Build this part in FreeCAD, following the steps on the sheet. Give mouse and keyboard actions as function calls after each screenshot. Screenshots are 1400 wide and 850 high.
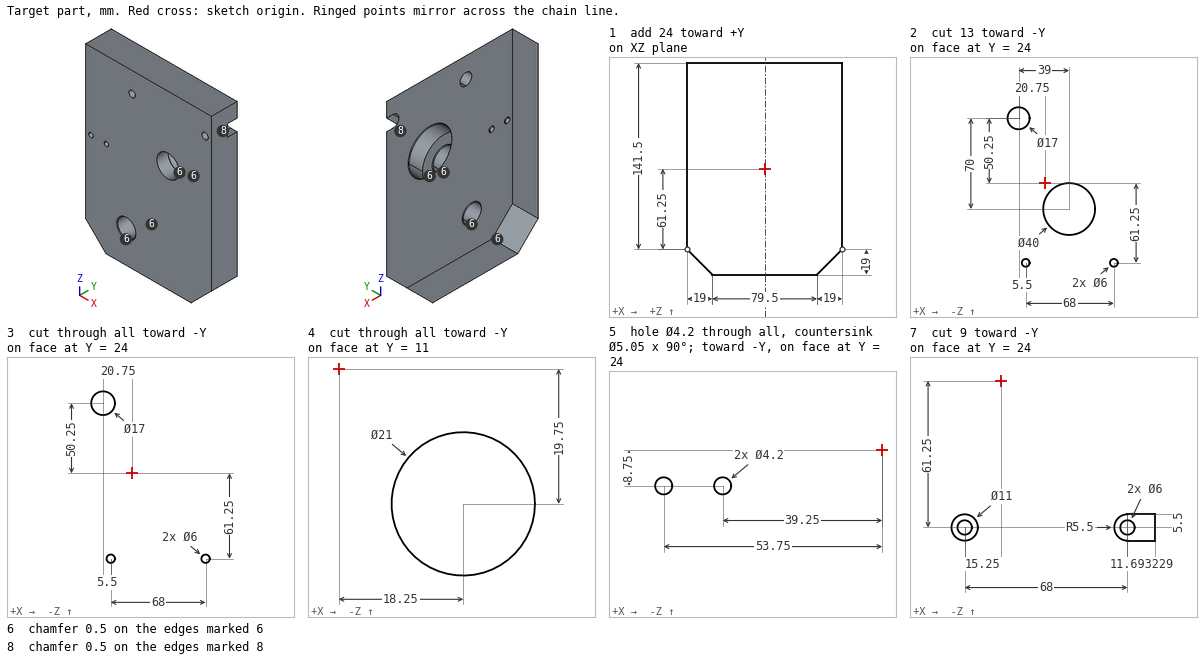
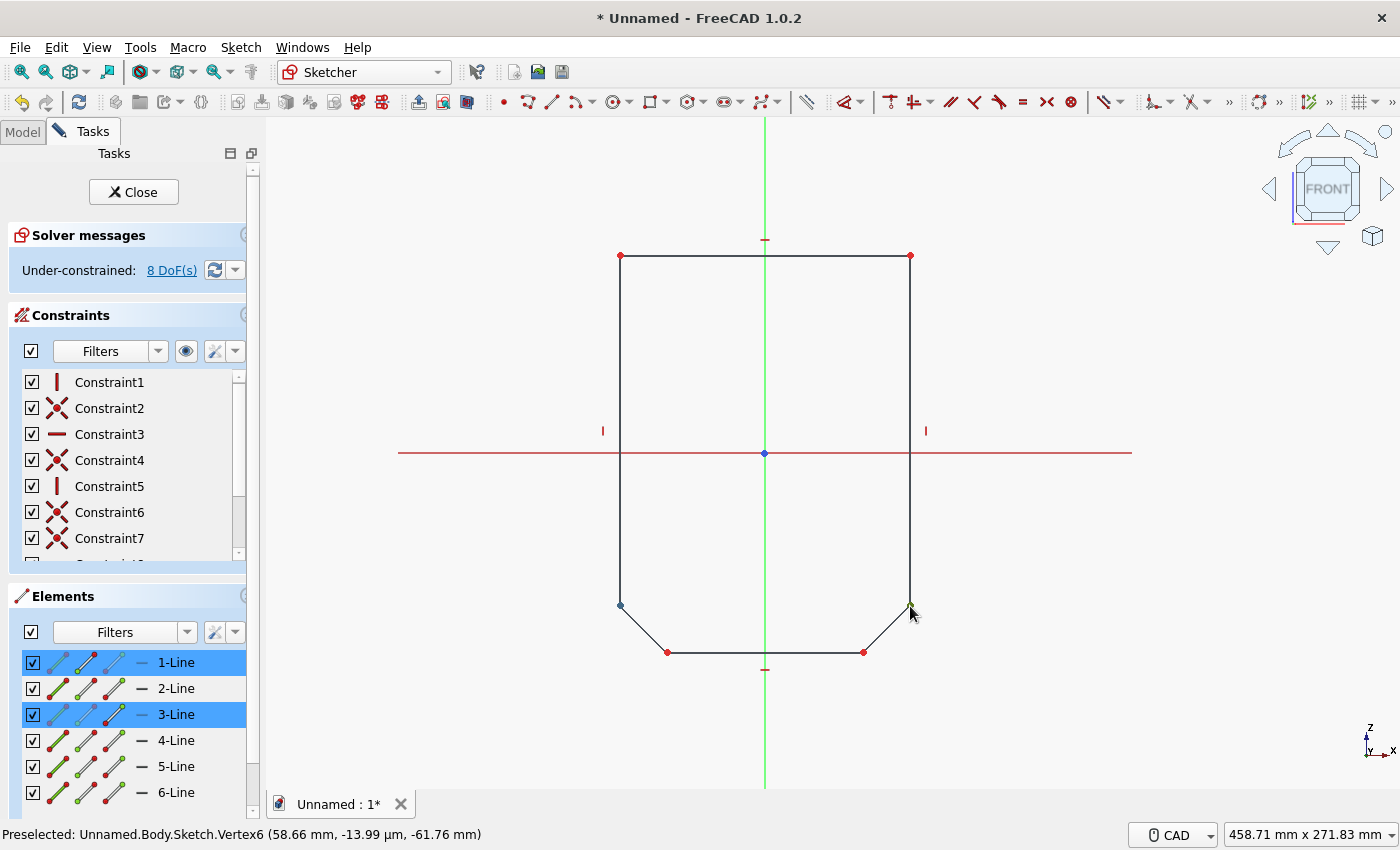
click(765, 717)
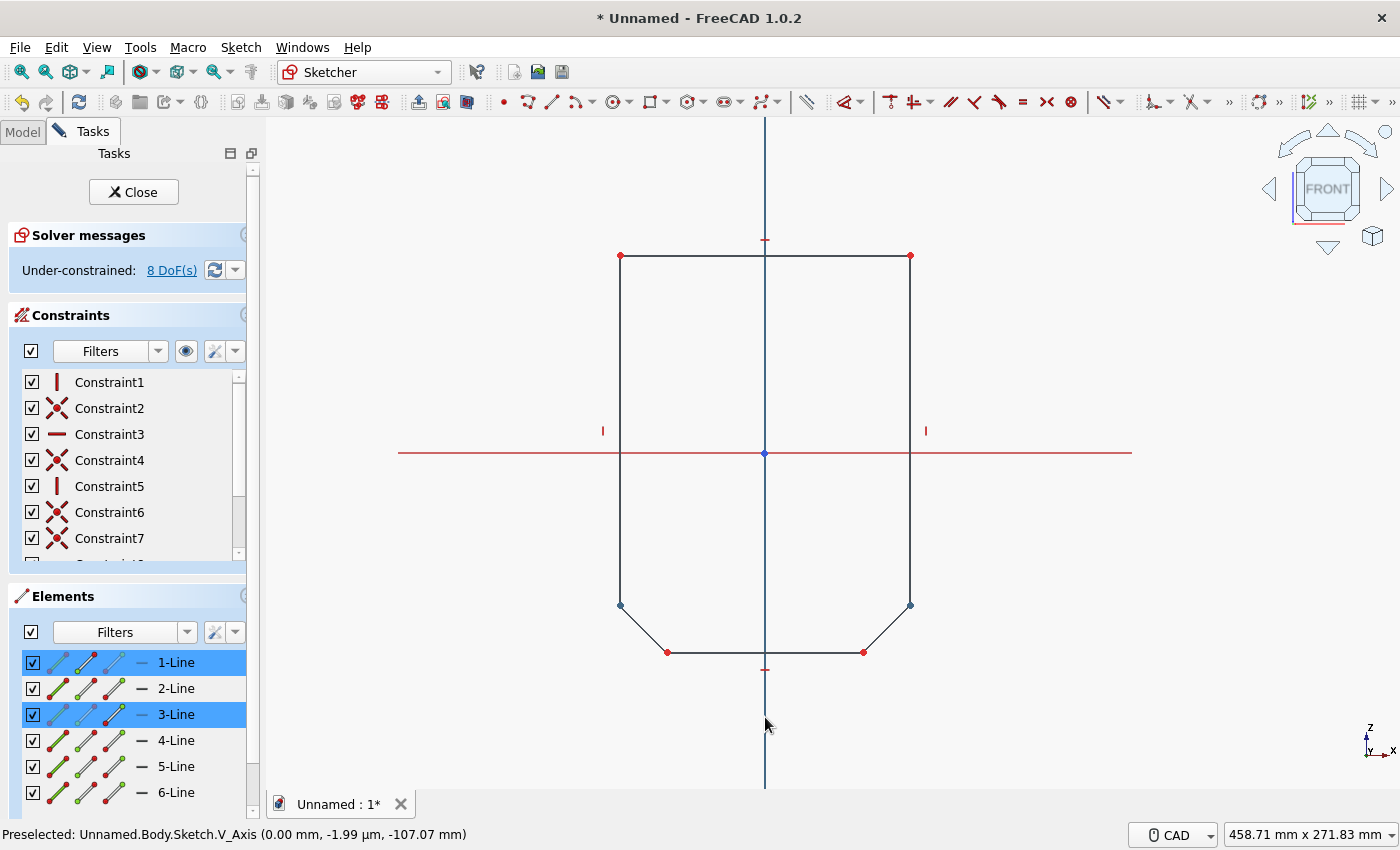
key(s)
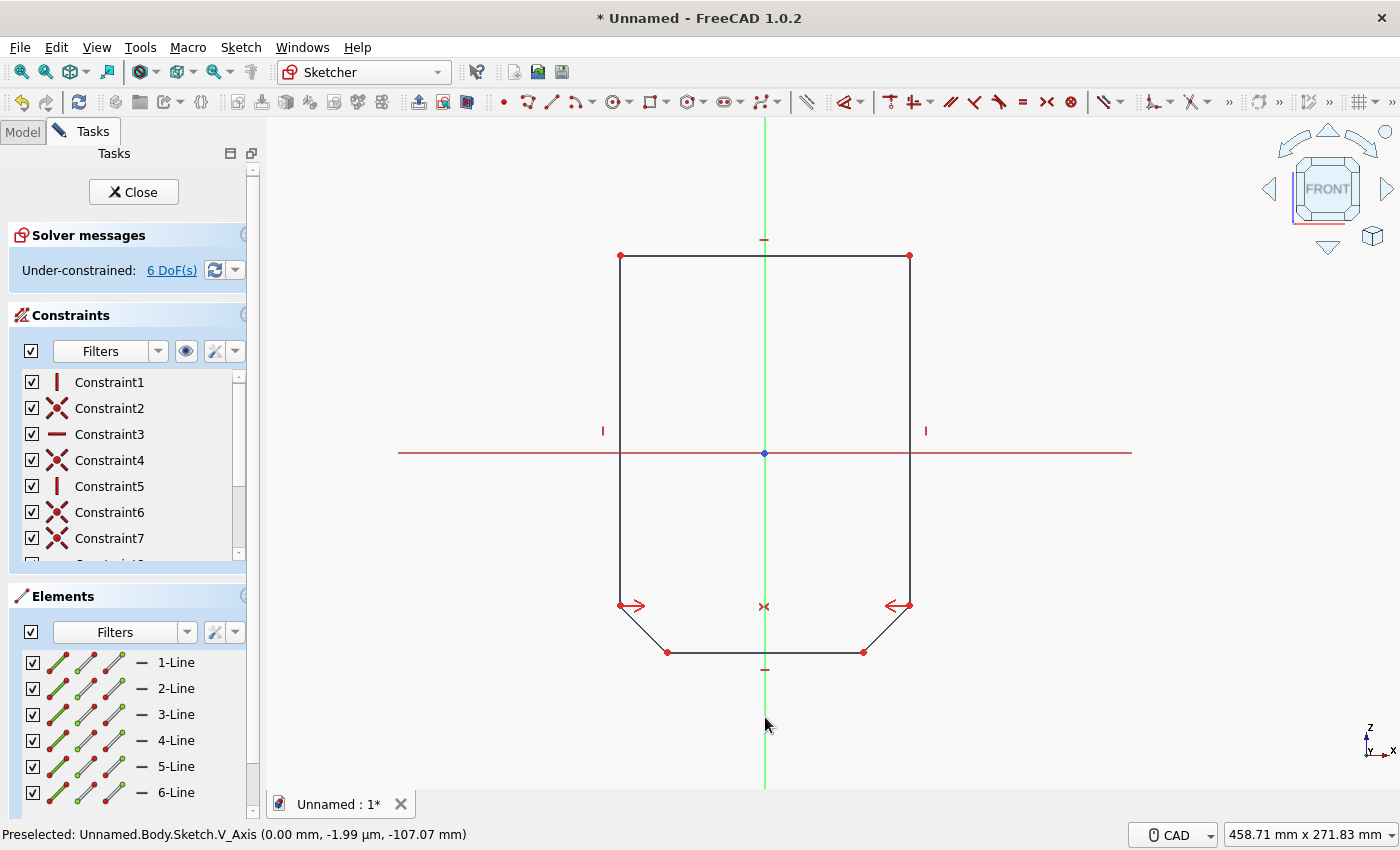
key(d)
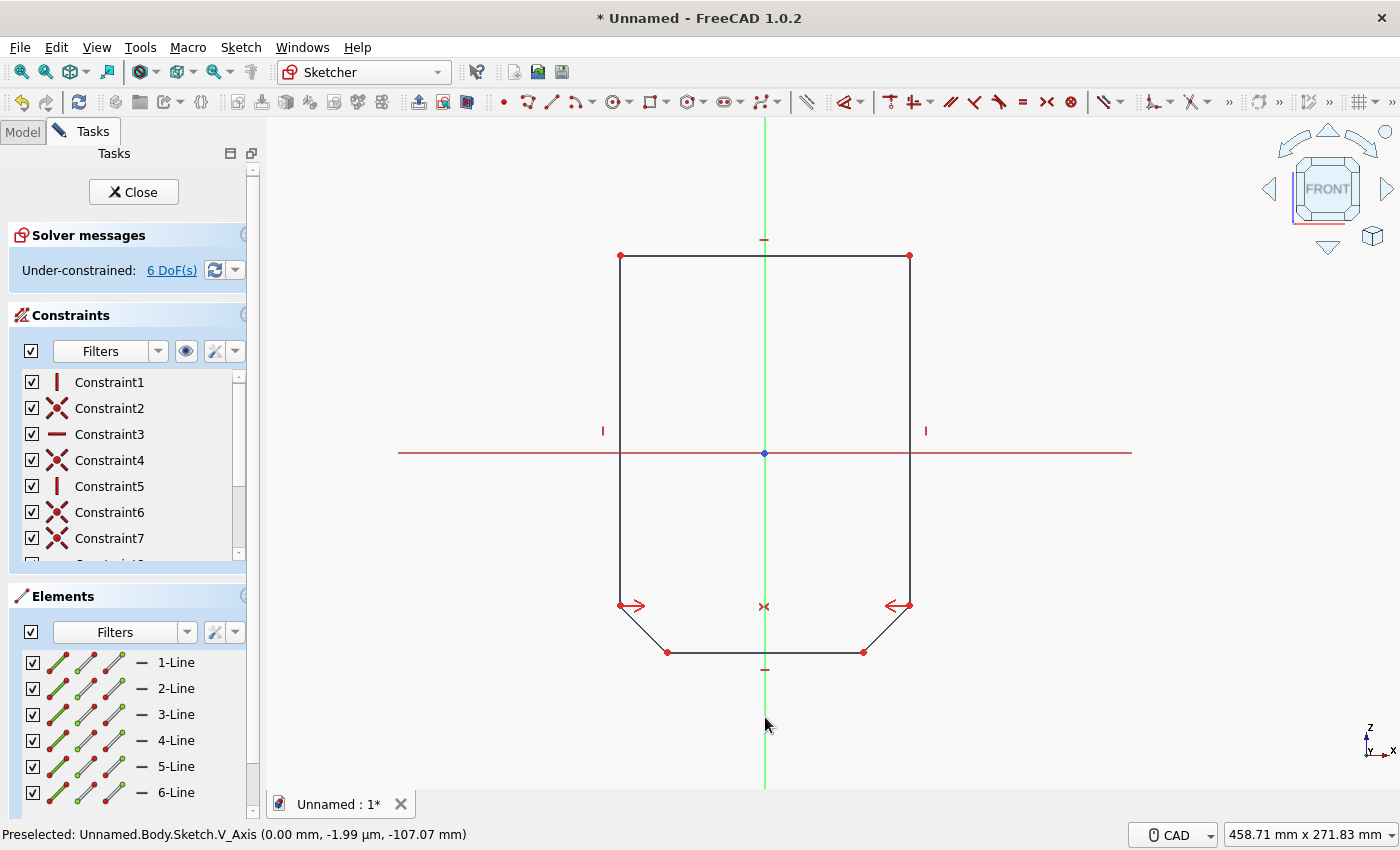
click(896, 620)
click(886, 687)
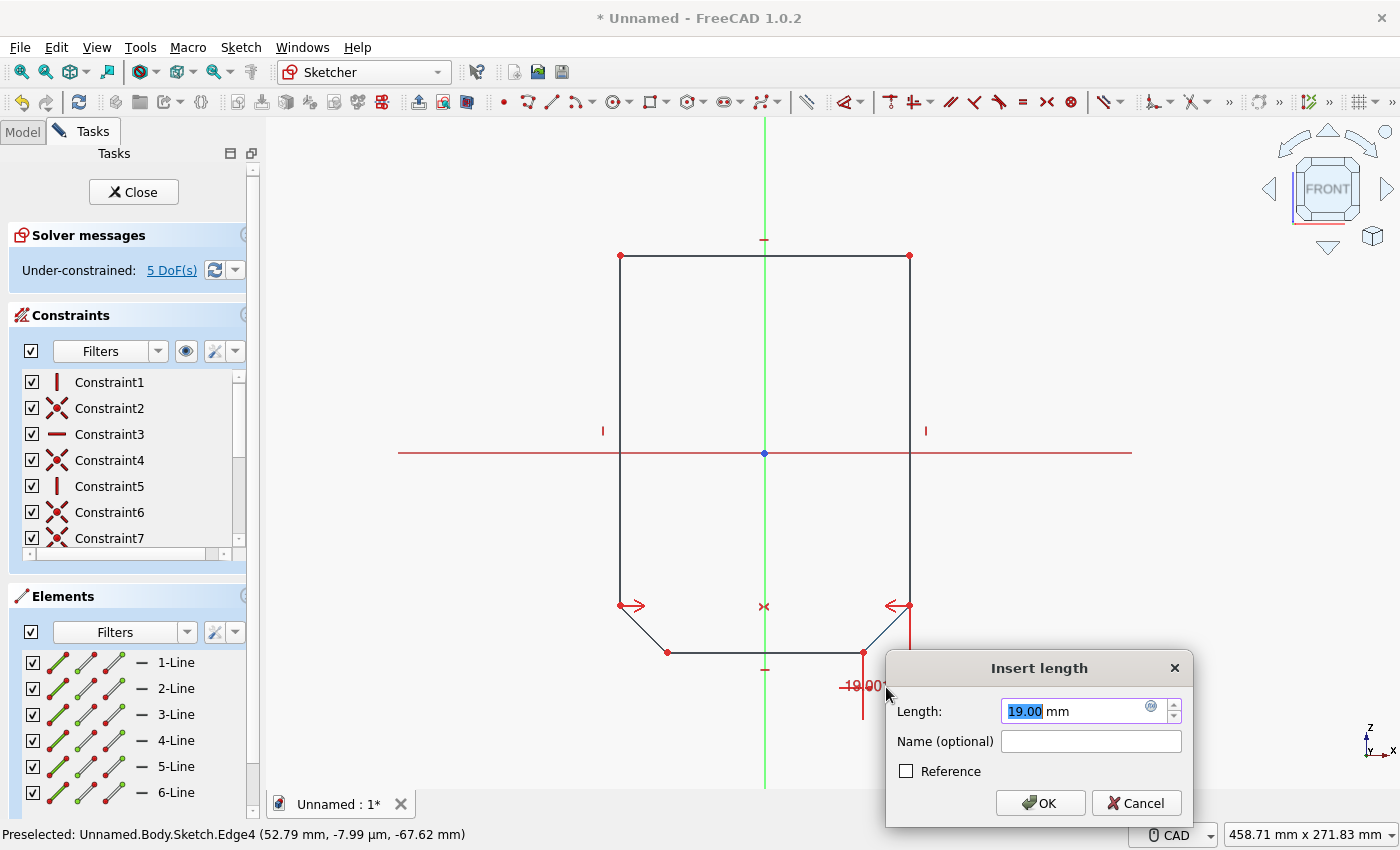
text(19)
key(Return)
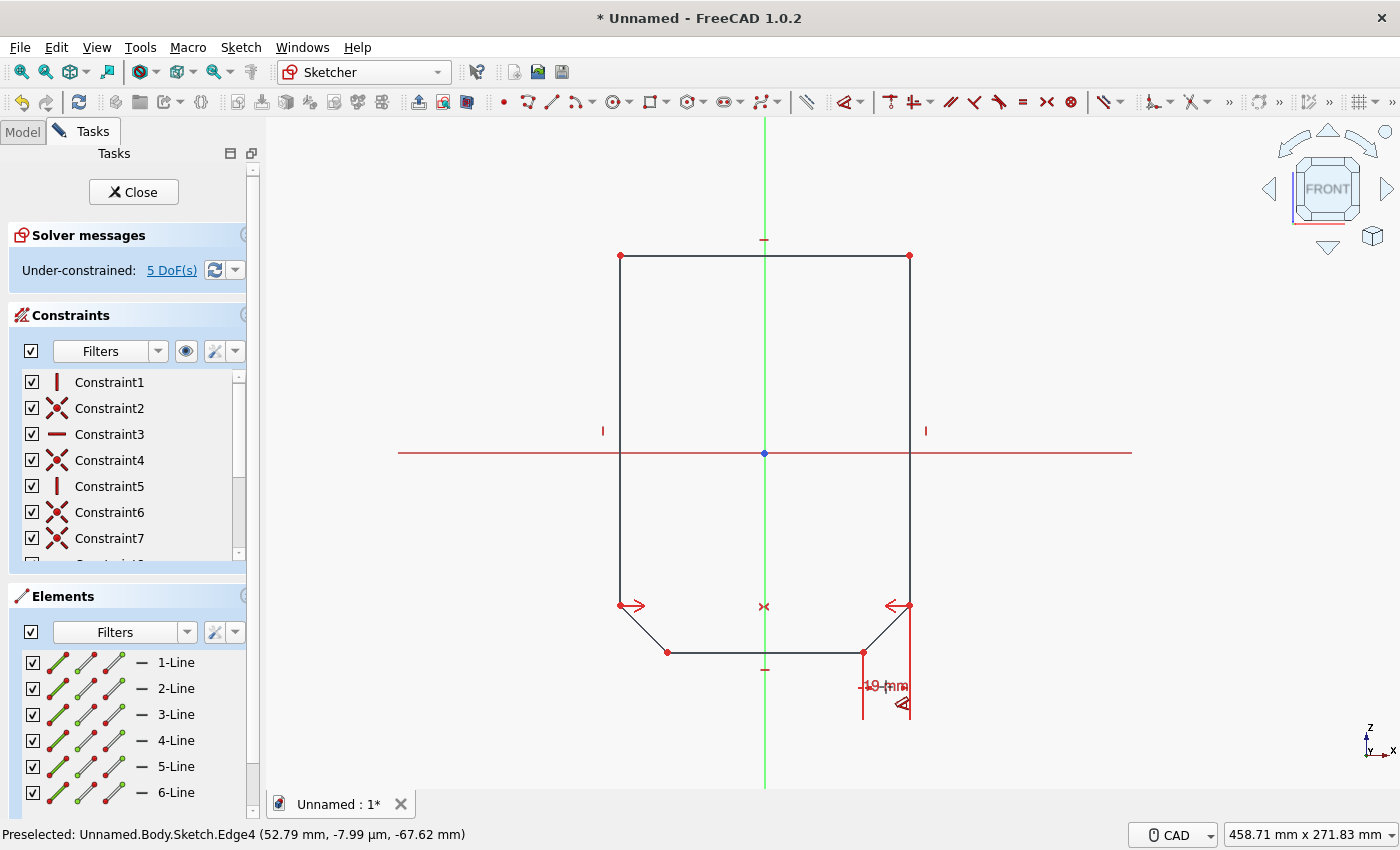
click(896, 620)
click(944, 629)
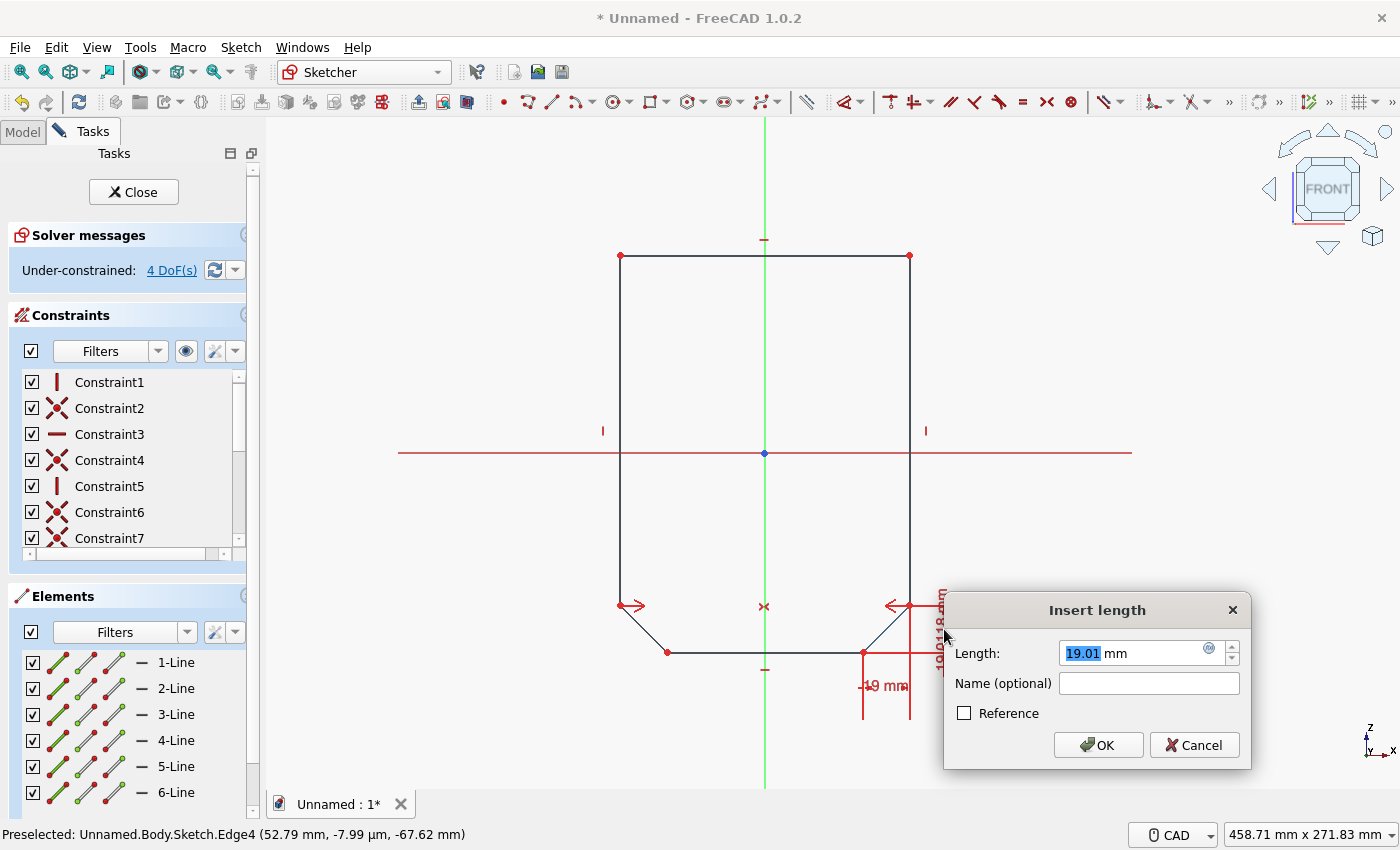
text(19)
key(Return)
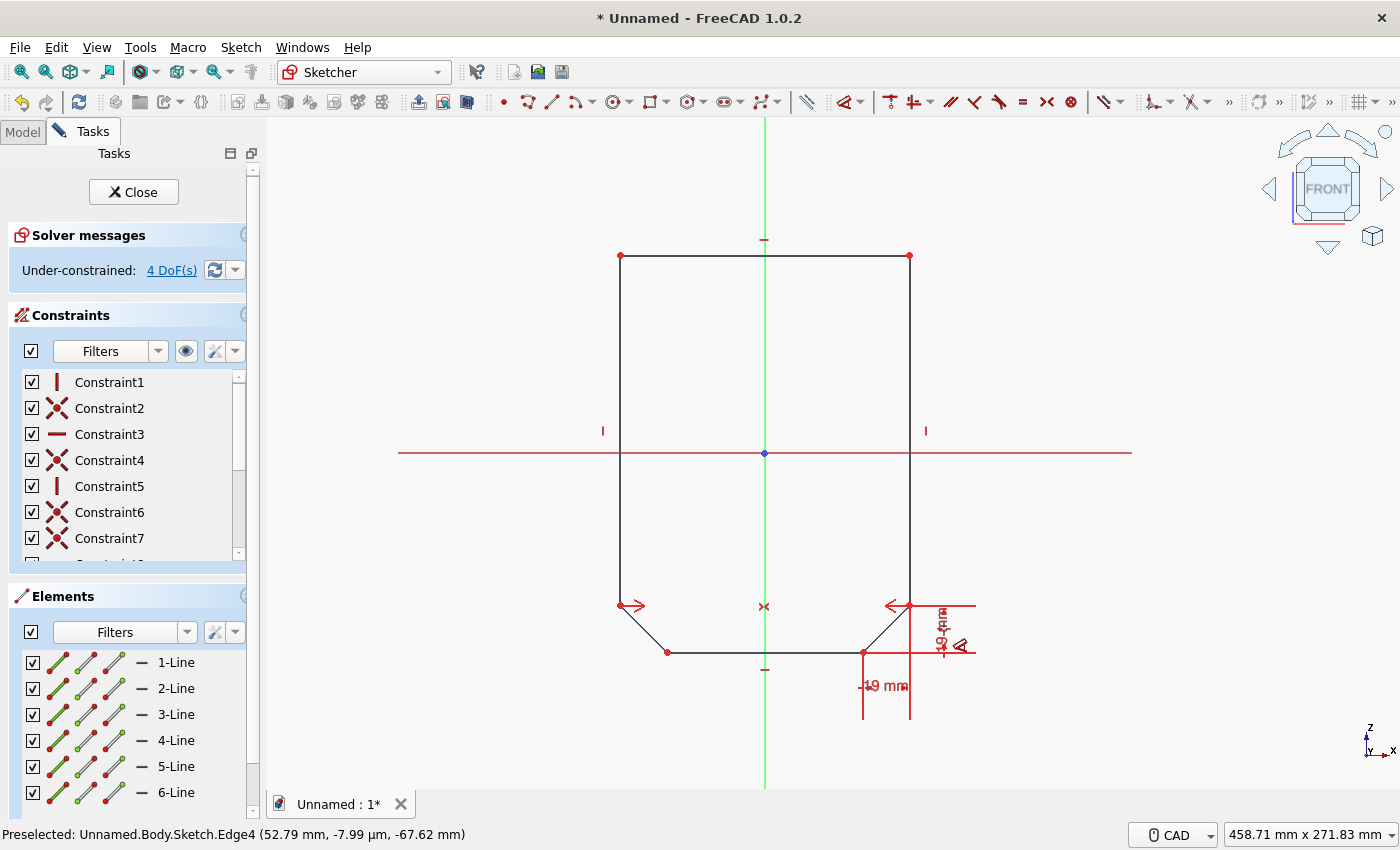
click(653, 639)
click(644, 687)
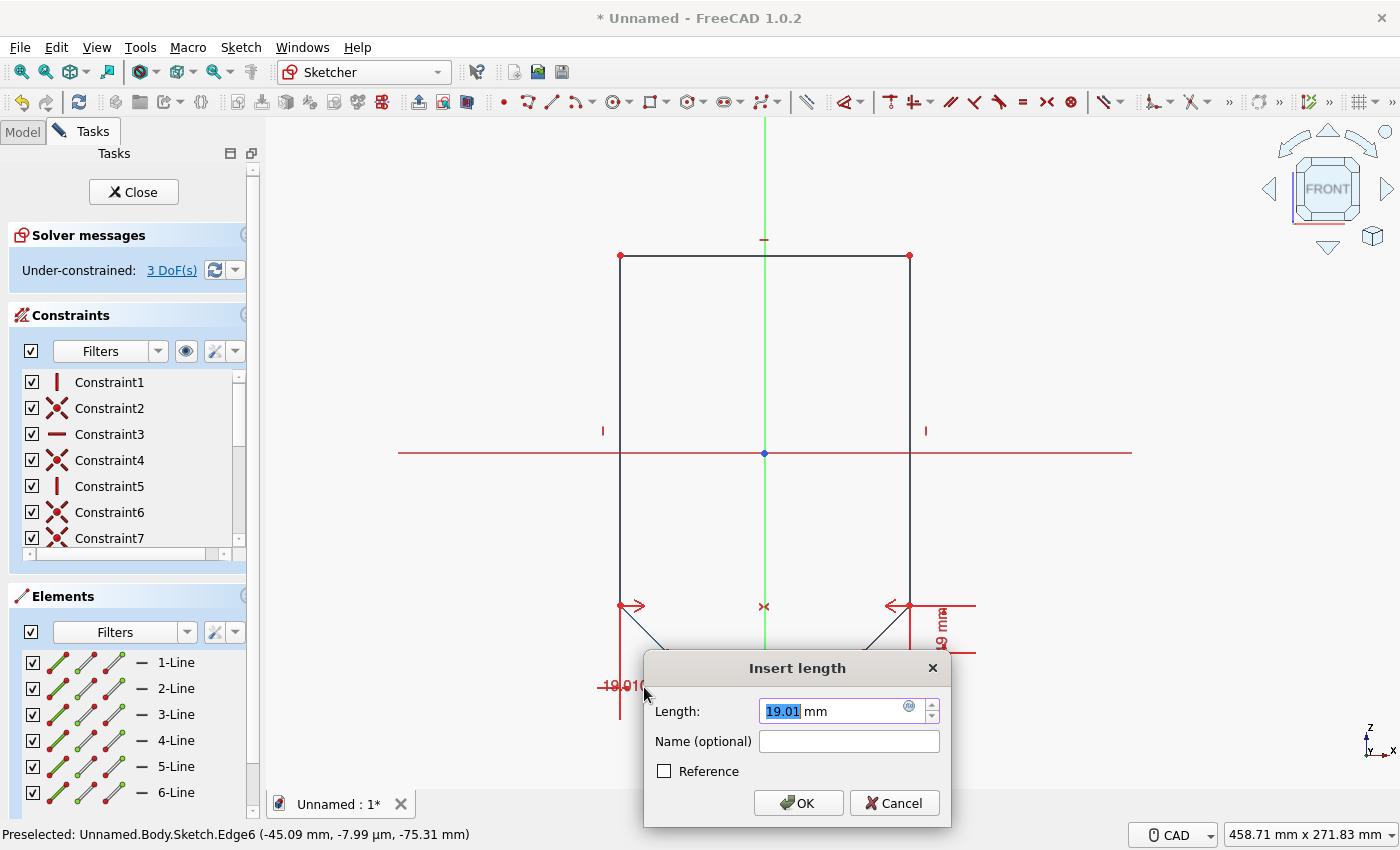
text(19)
key(Return)